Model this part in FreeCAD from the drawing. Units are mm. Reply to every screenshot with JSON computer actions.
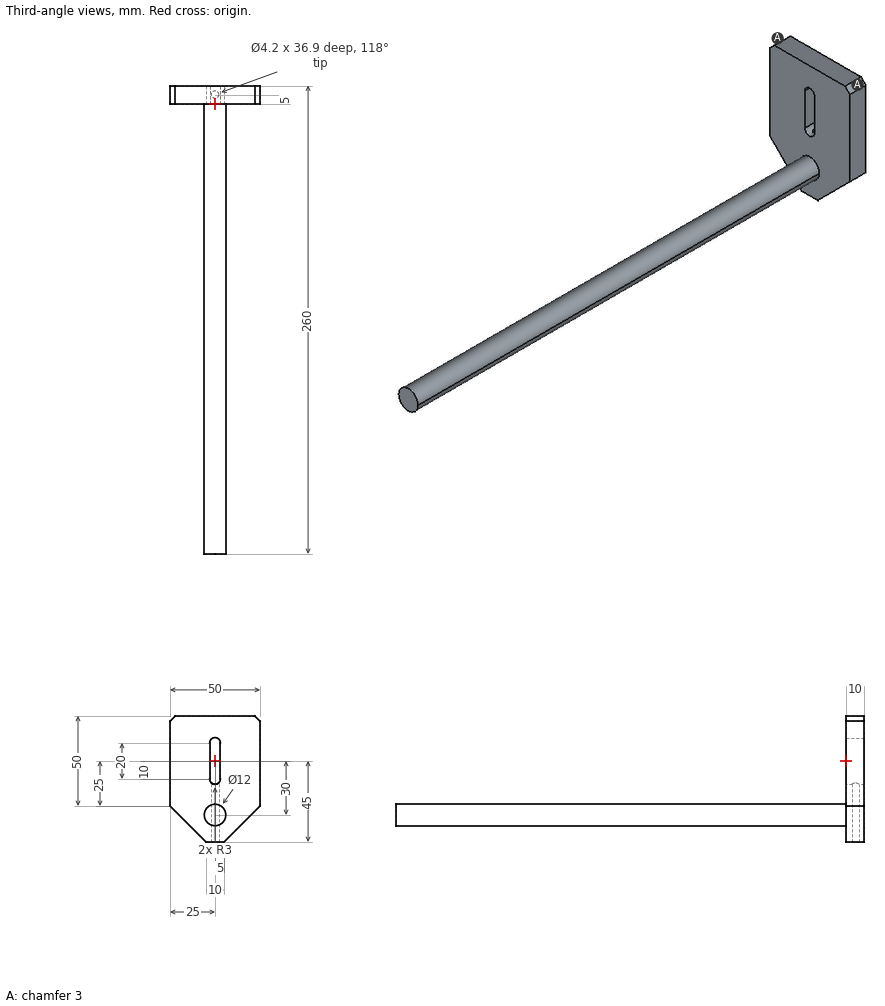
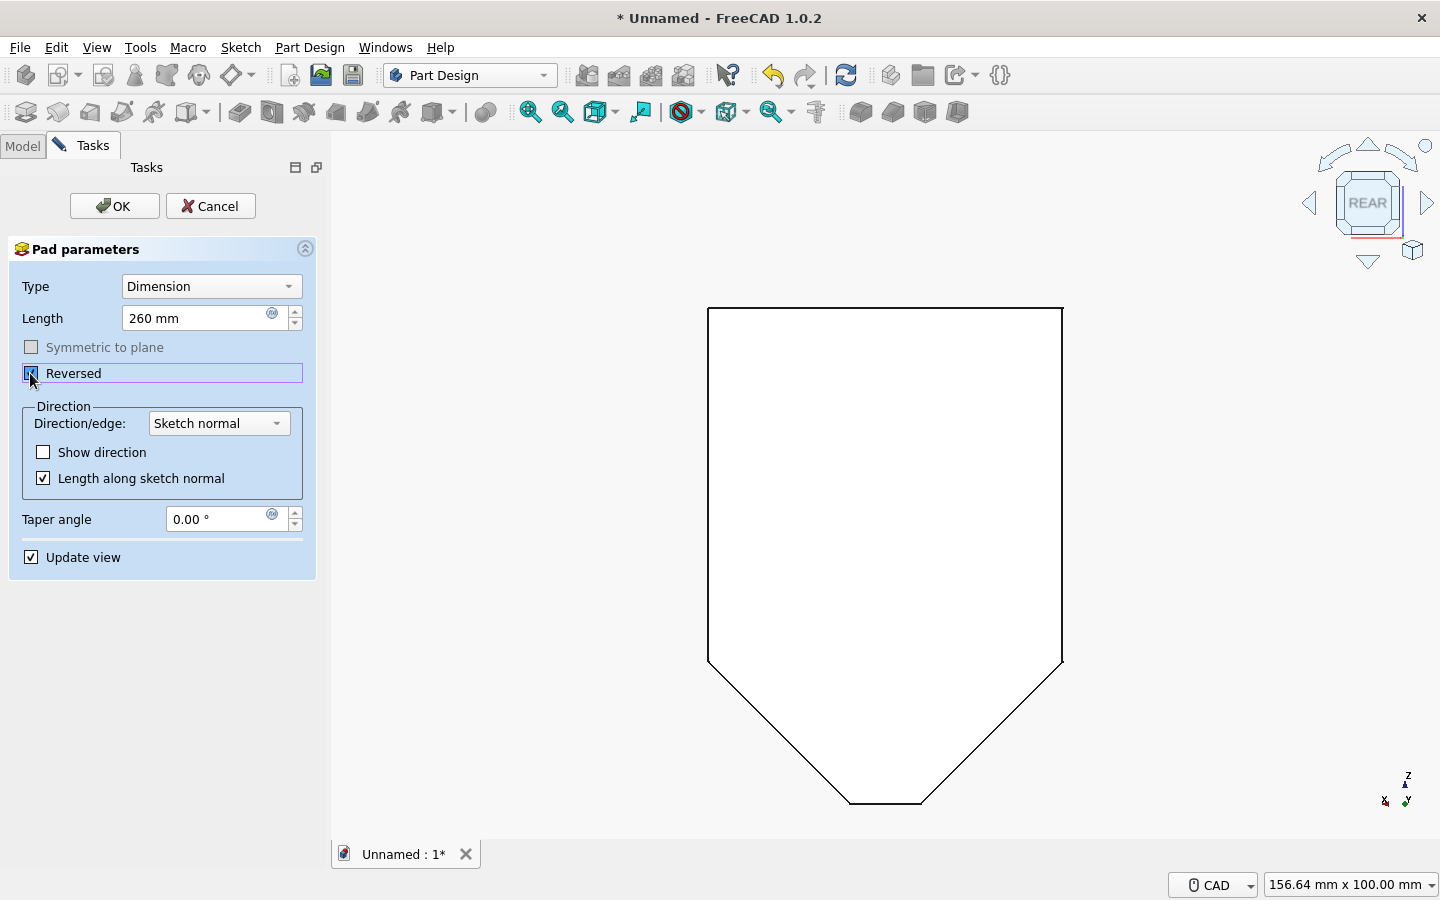
{"action": "left_click", "coordinate": [115, 206]}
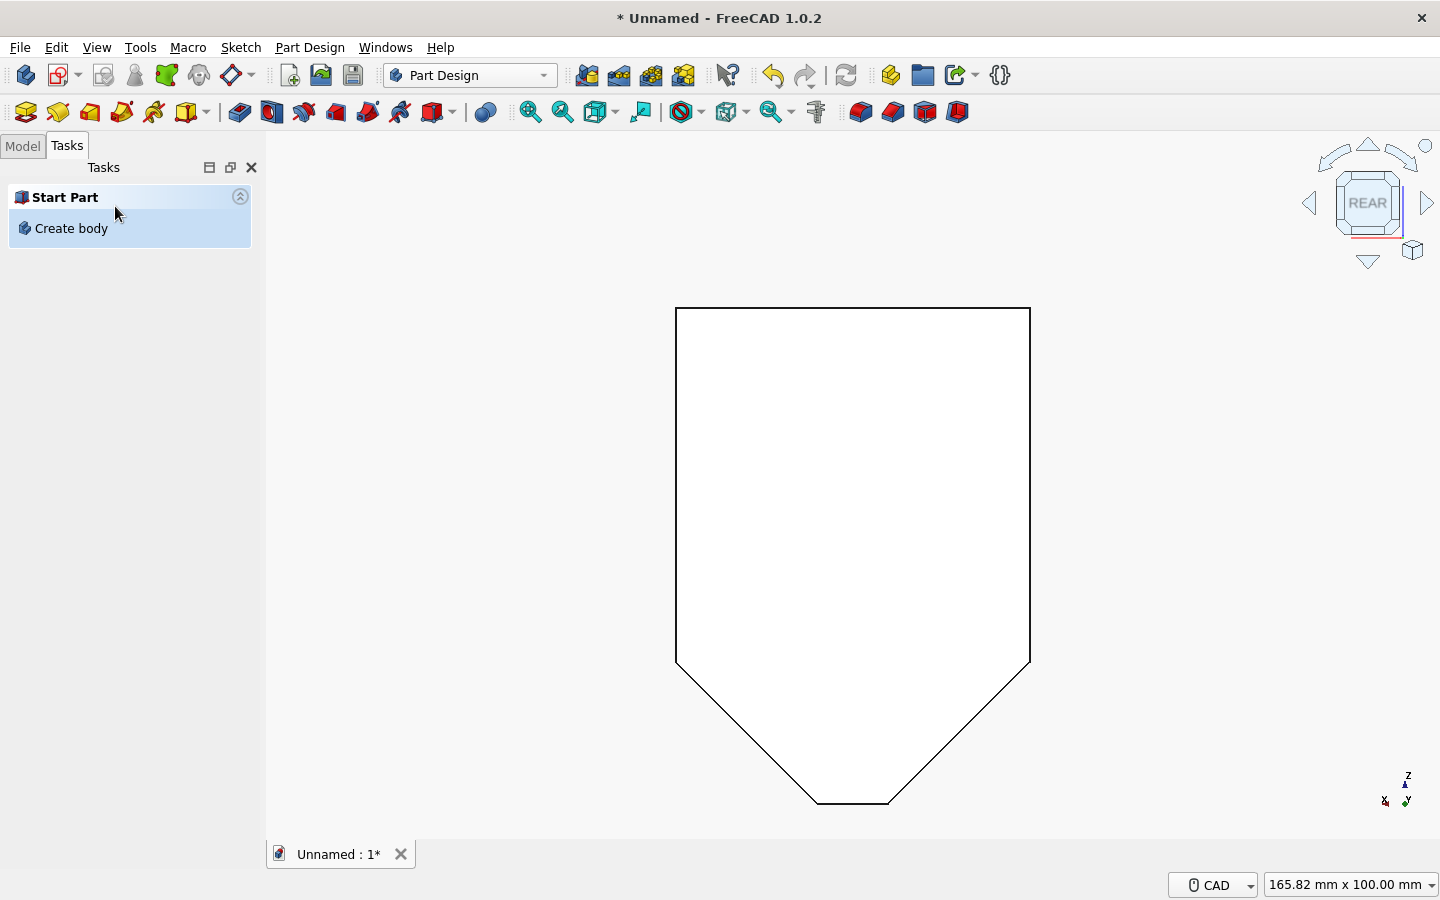
{"action": "left_click", "coordinate": [58, 76]}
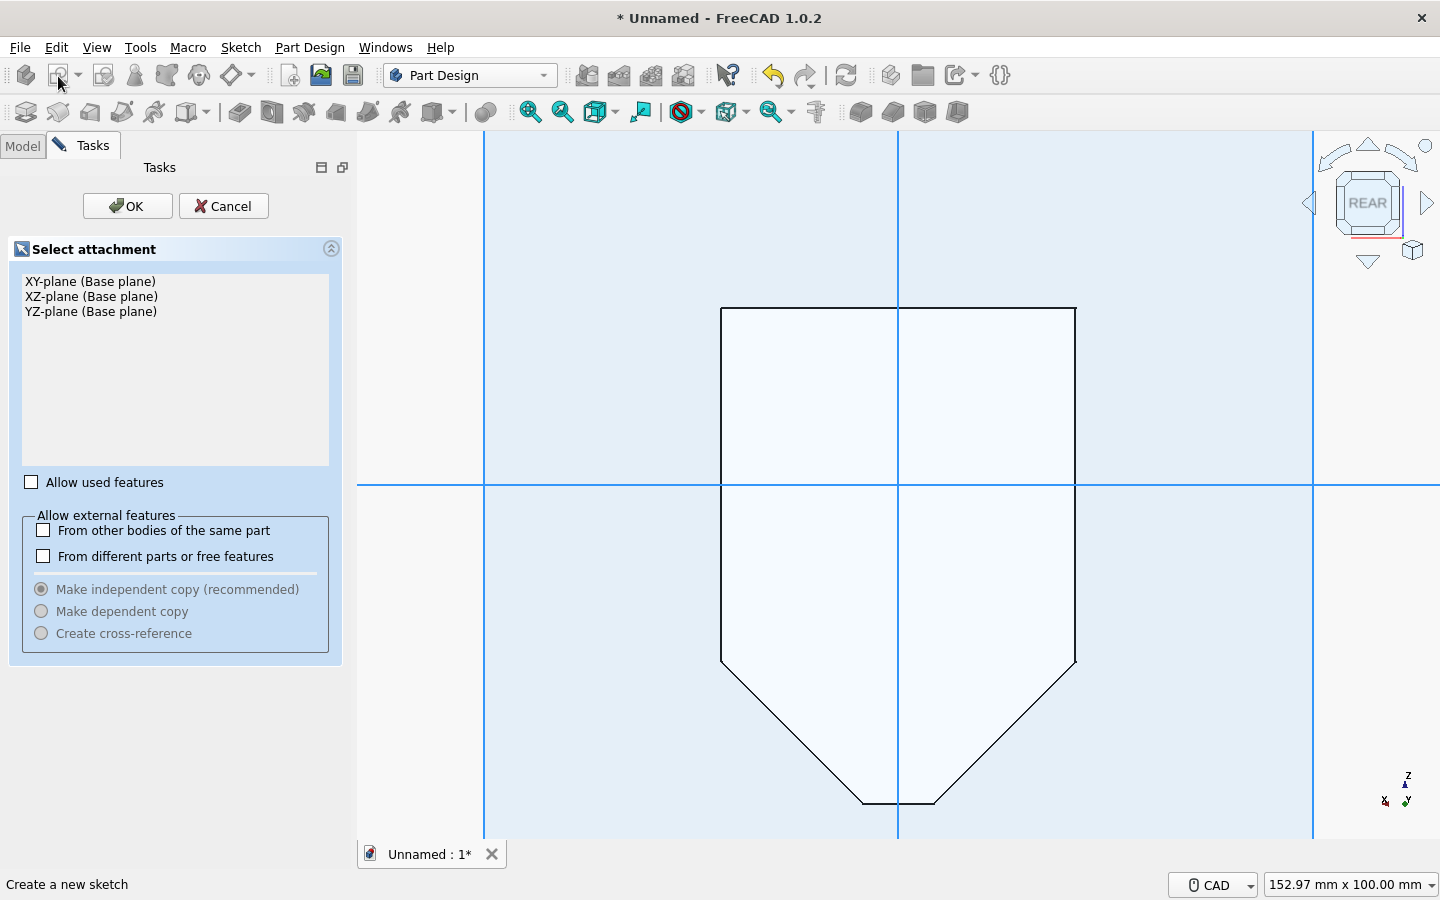
{"action": "left_click", "coordinate": [82, 296]}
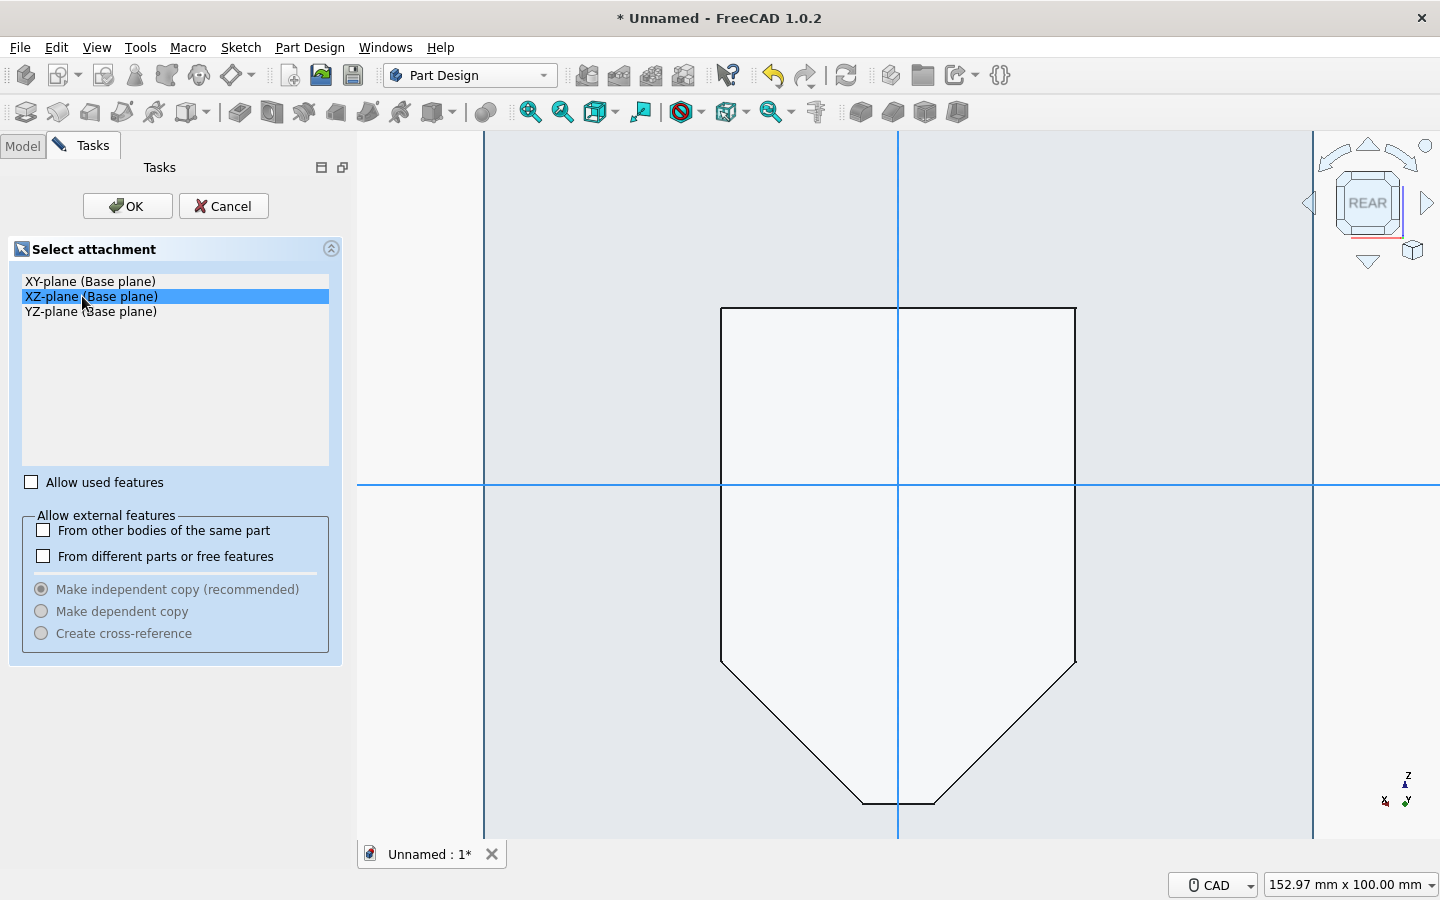
{"action": "left_click", "coordinate": [128, 206]}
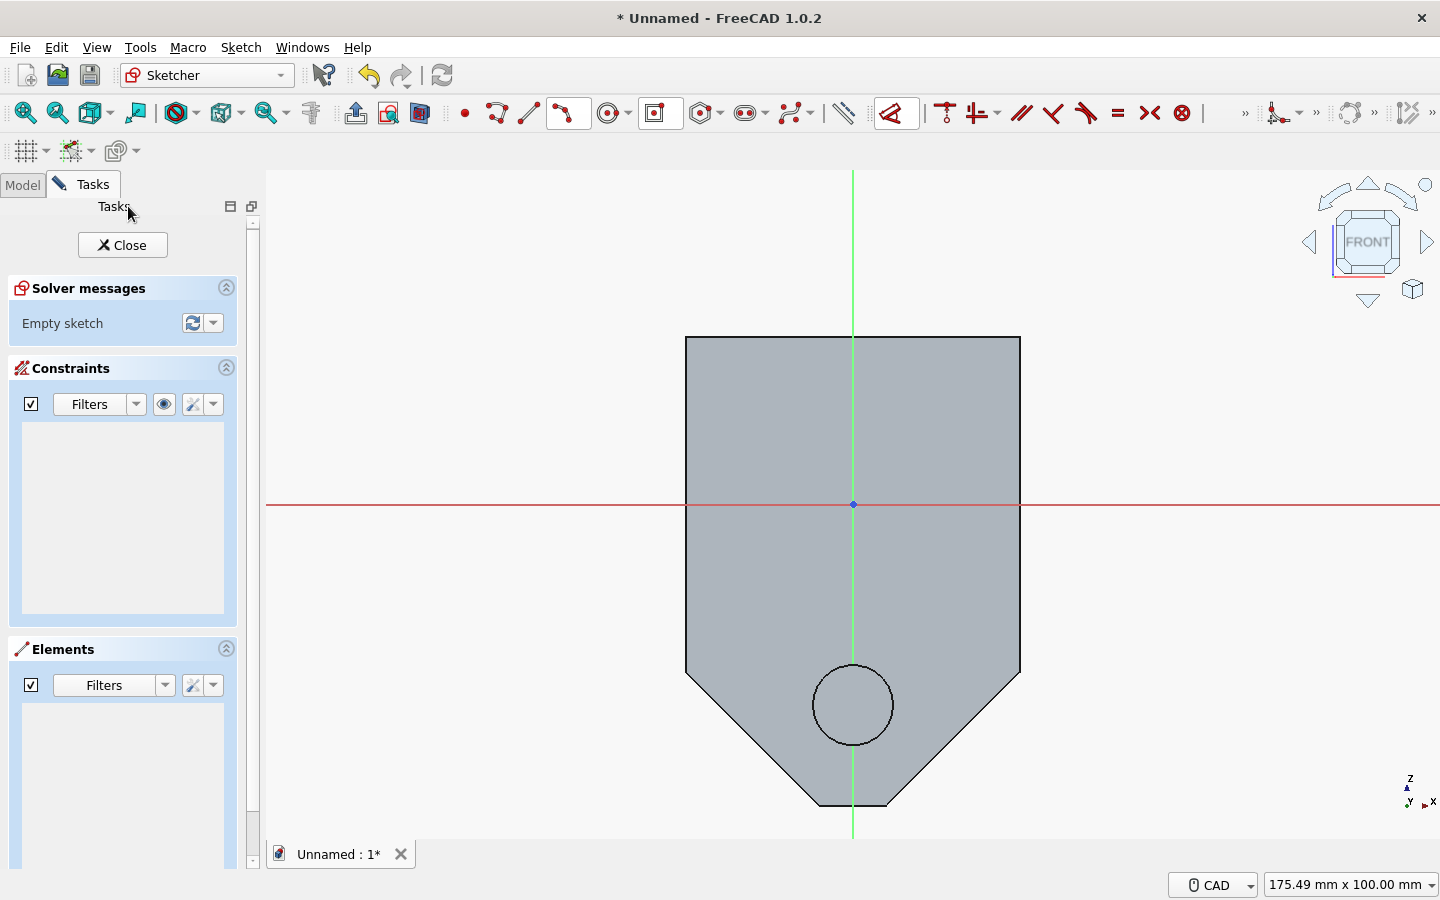
{"action": "left_click", "coordinate": [420, 114]}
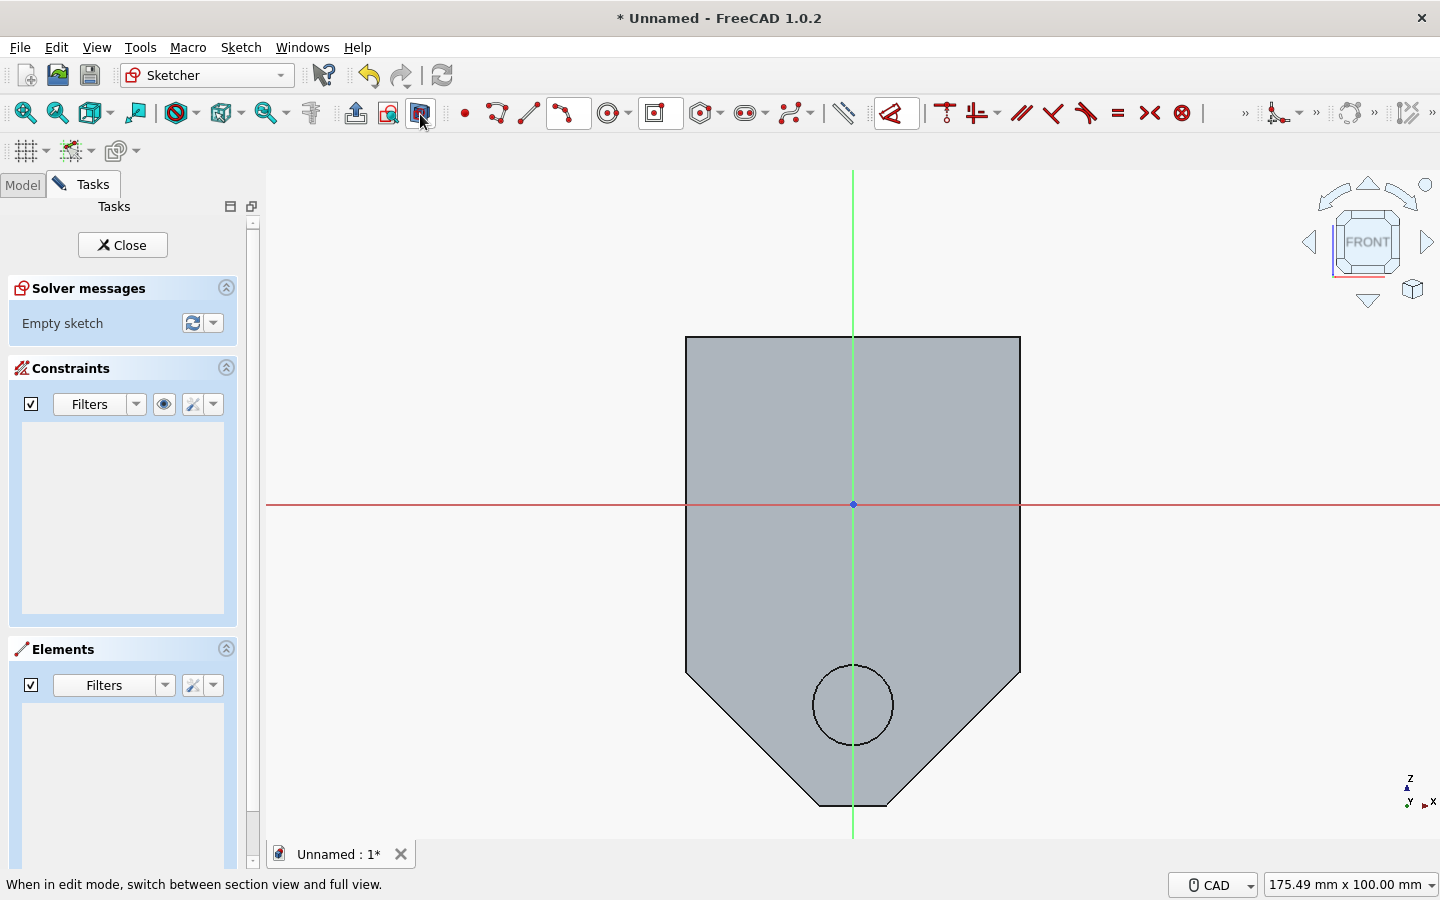
{"action": "scroll", "coordinate": [893, 505], "scroll_direction": "up", "scroll_amount": 5}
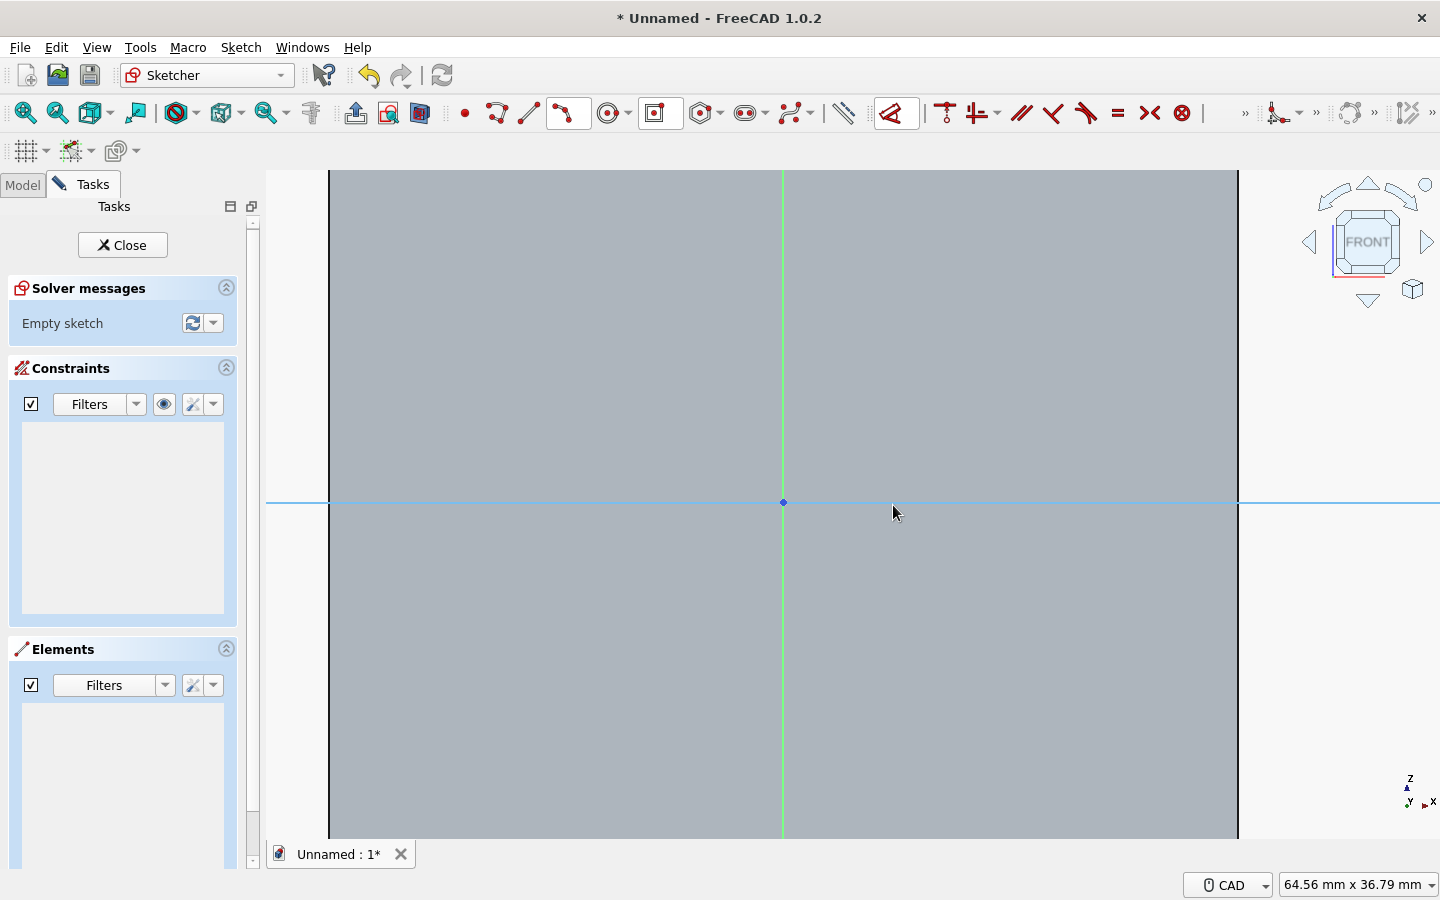
{"action": "left_click", "coordinate": [746, 114]}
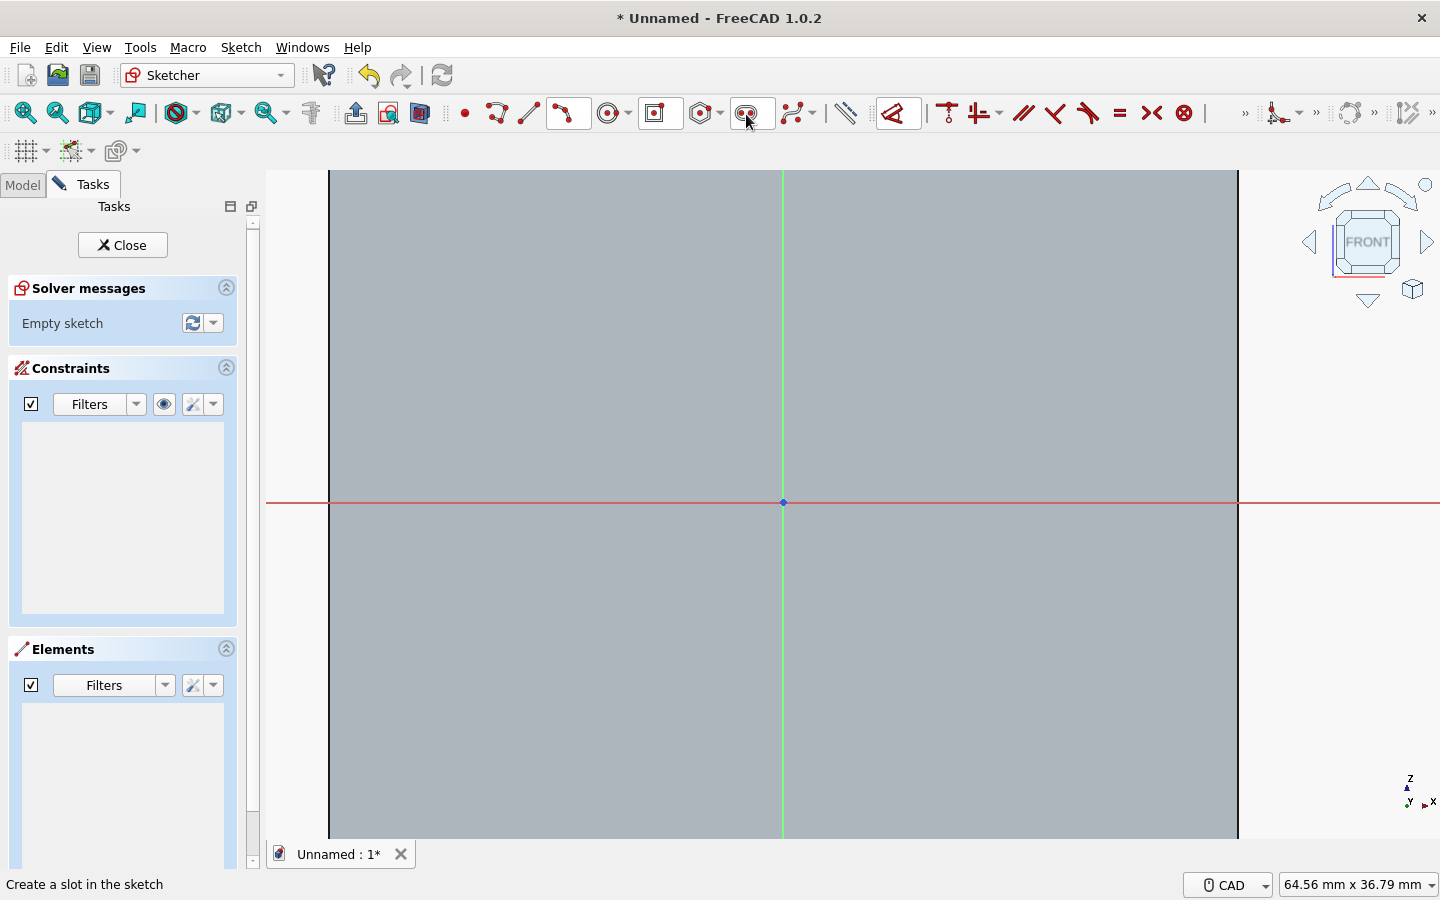
{"action": "left_click", "coordinate": [783, 685]}